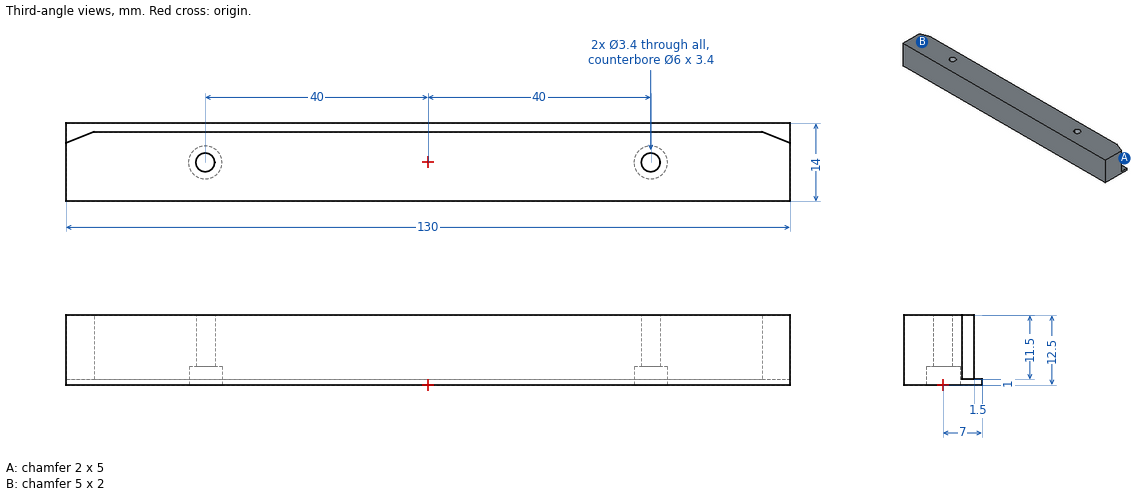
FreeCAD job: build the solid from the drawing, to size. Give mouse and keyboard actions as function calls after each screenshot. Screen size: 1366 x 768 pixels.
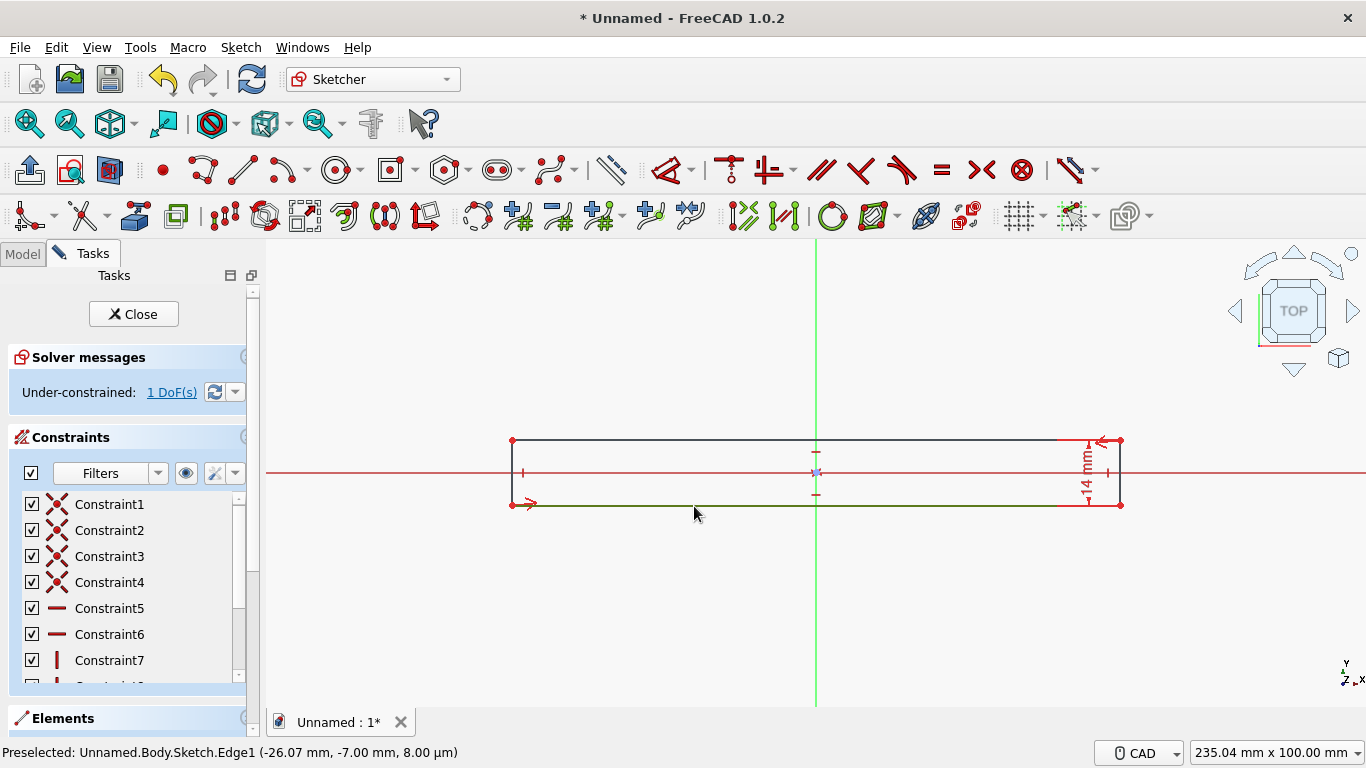
key(l)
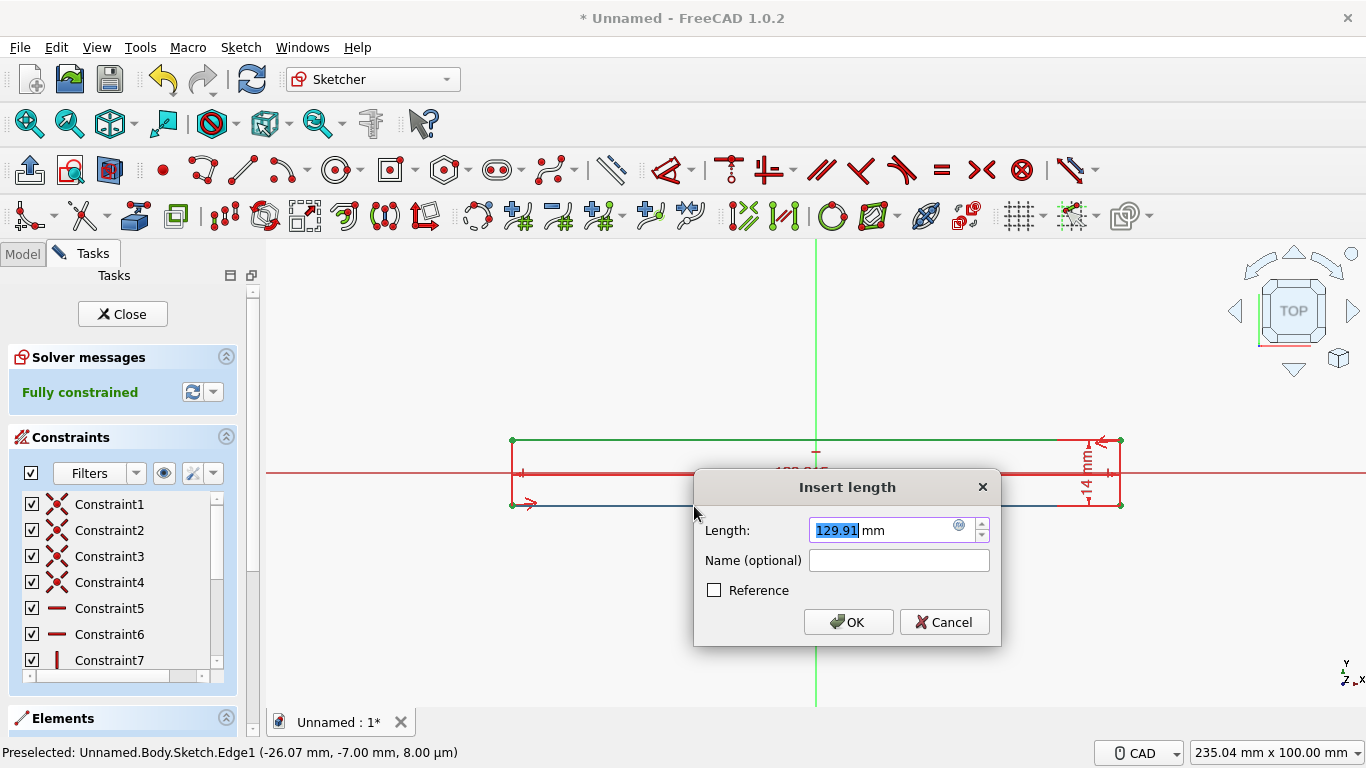
text(130)
key(Return)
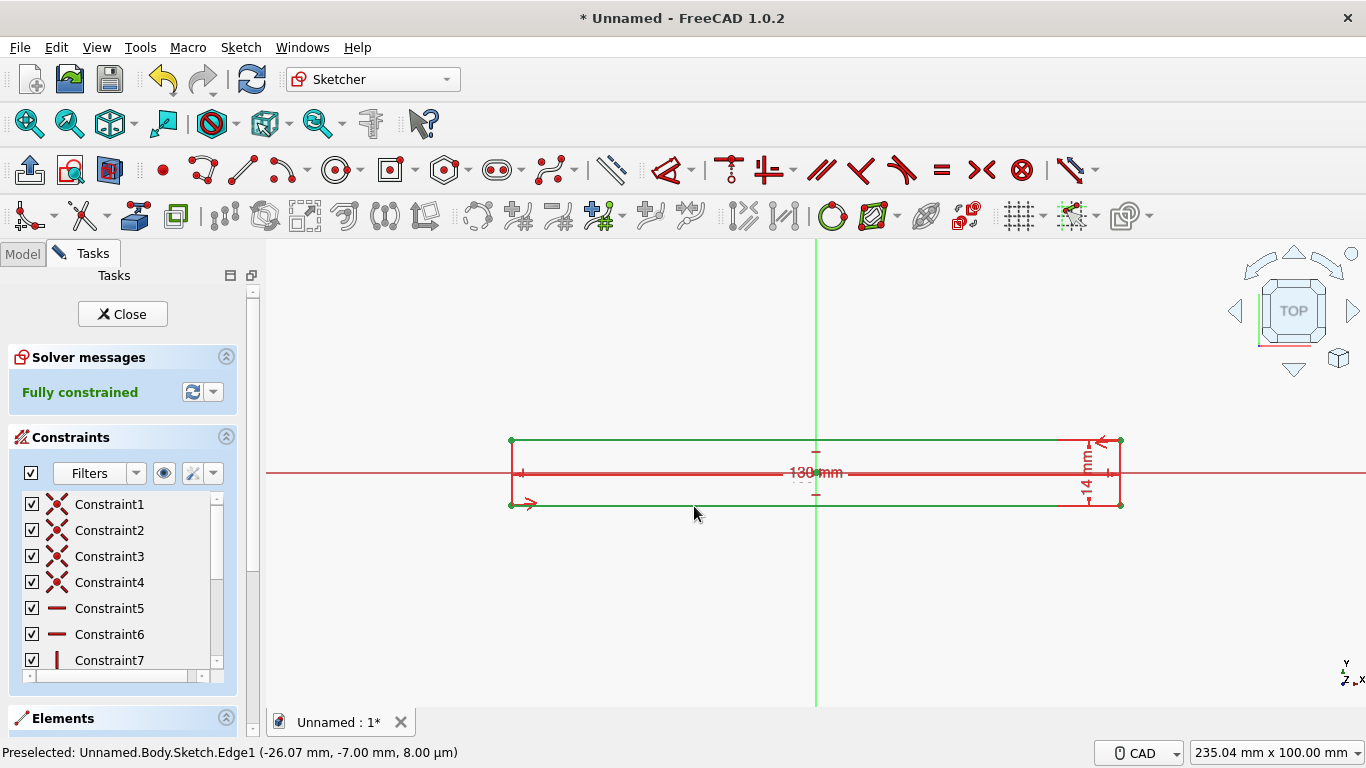
click(123, 314)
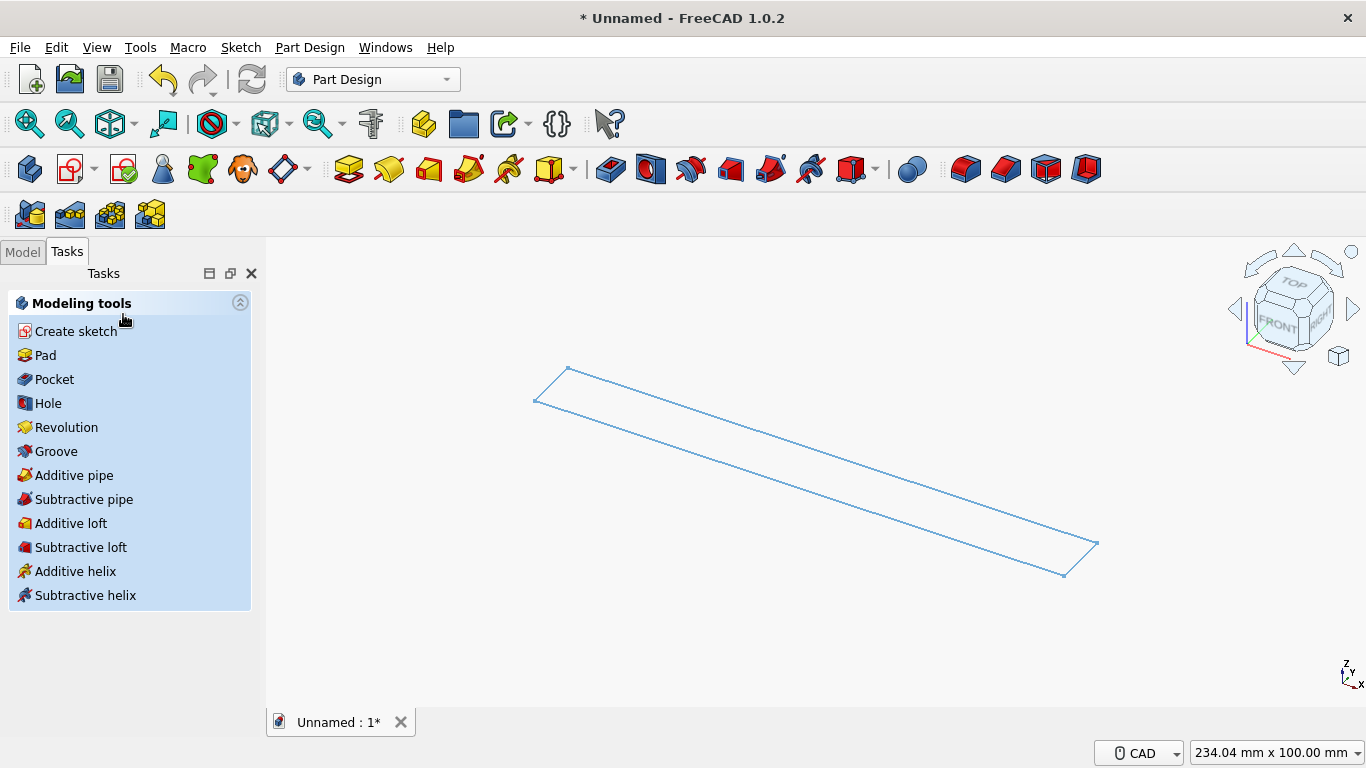
click(350, 170)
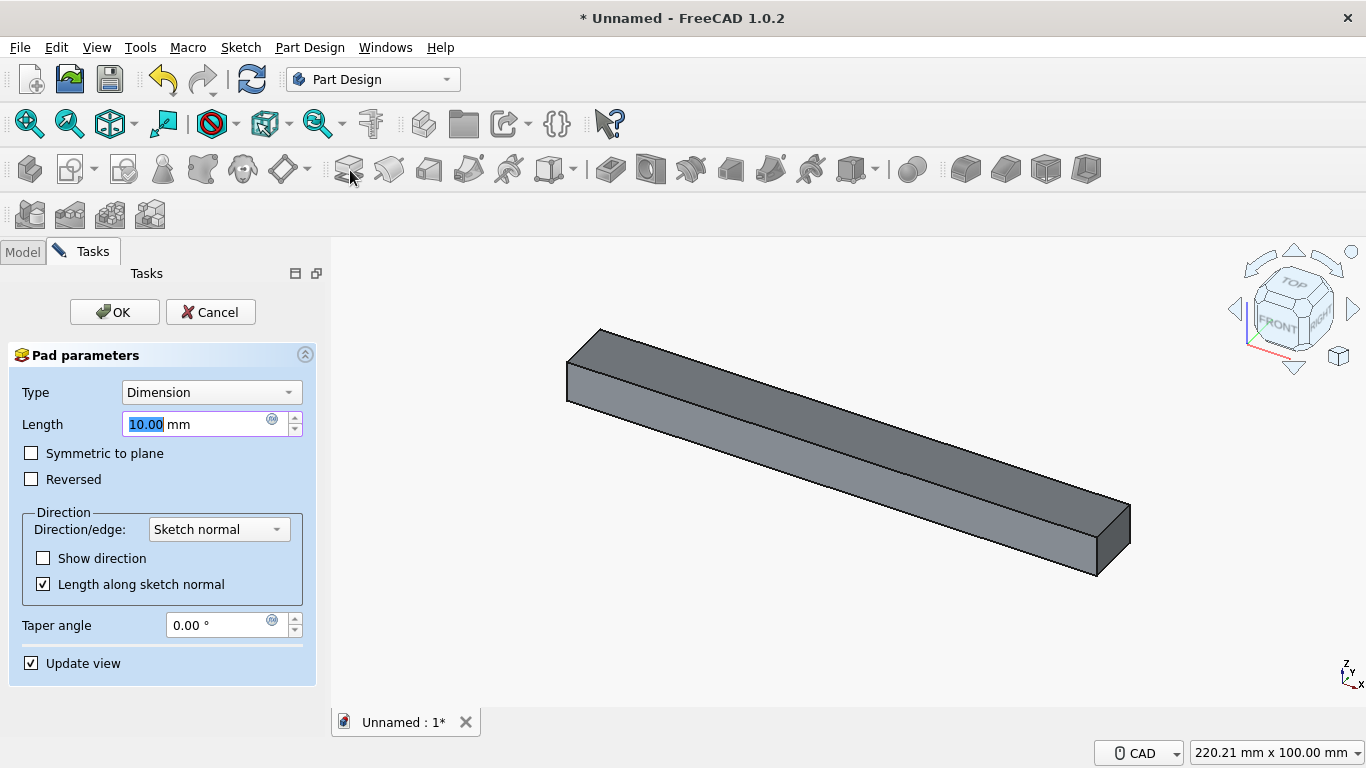
text(12.5)
key(Tab)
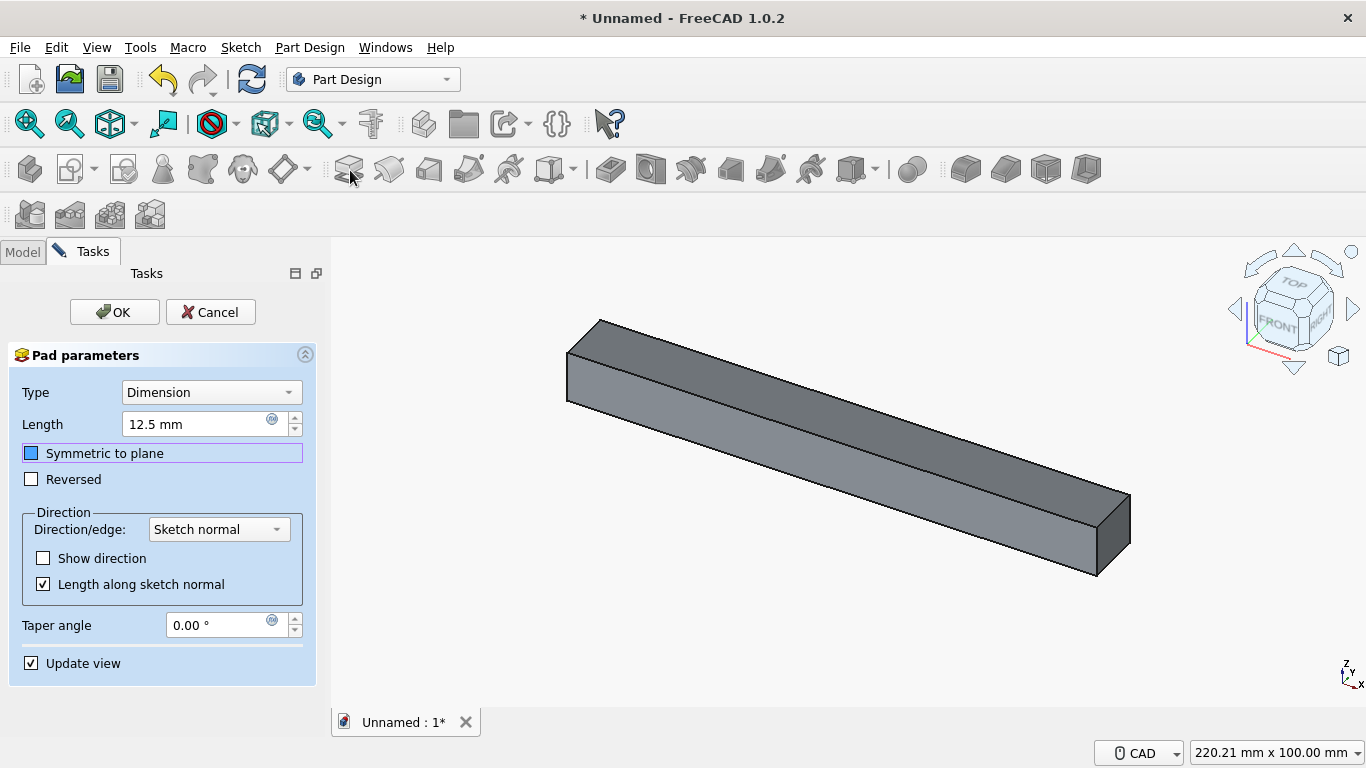
click(115, 312)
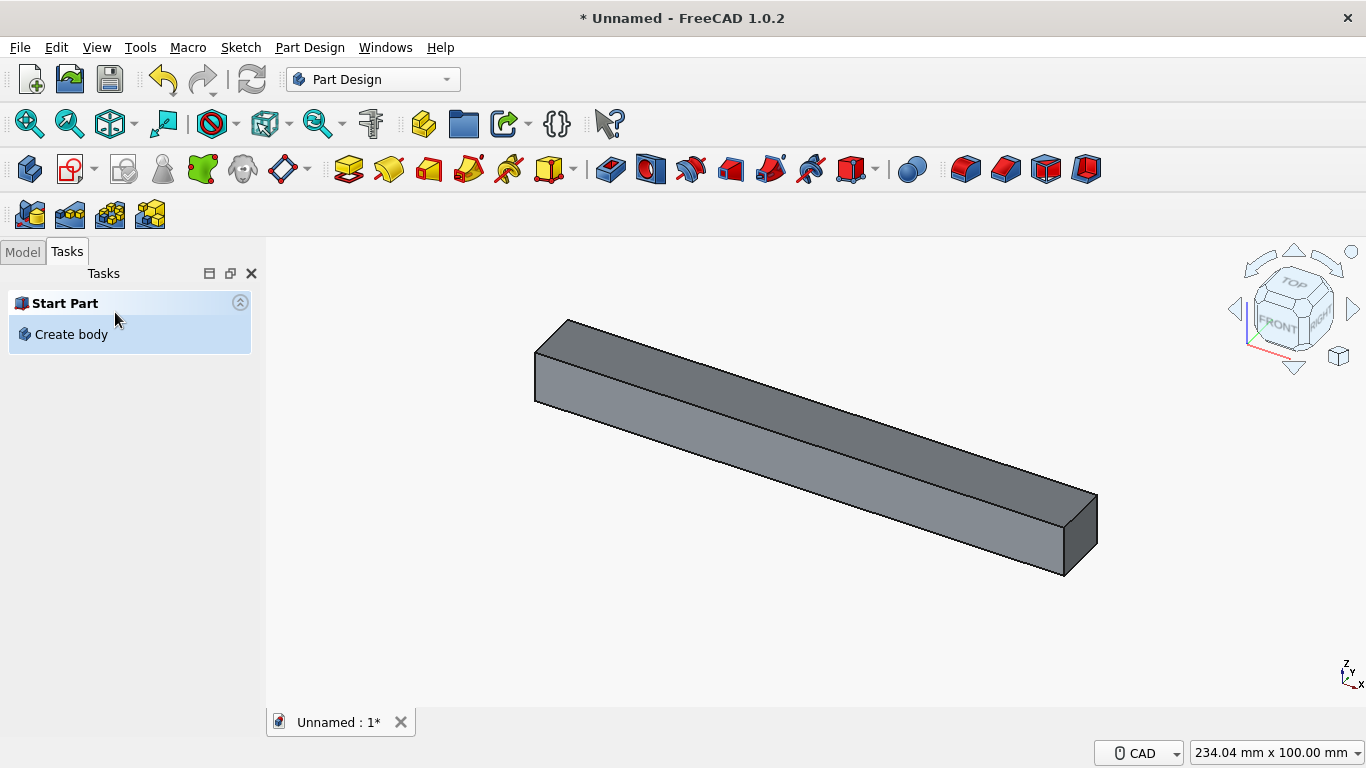
click(1081, 535)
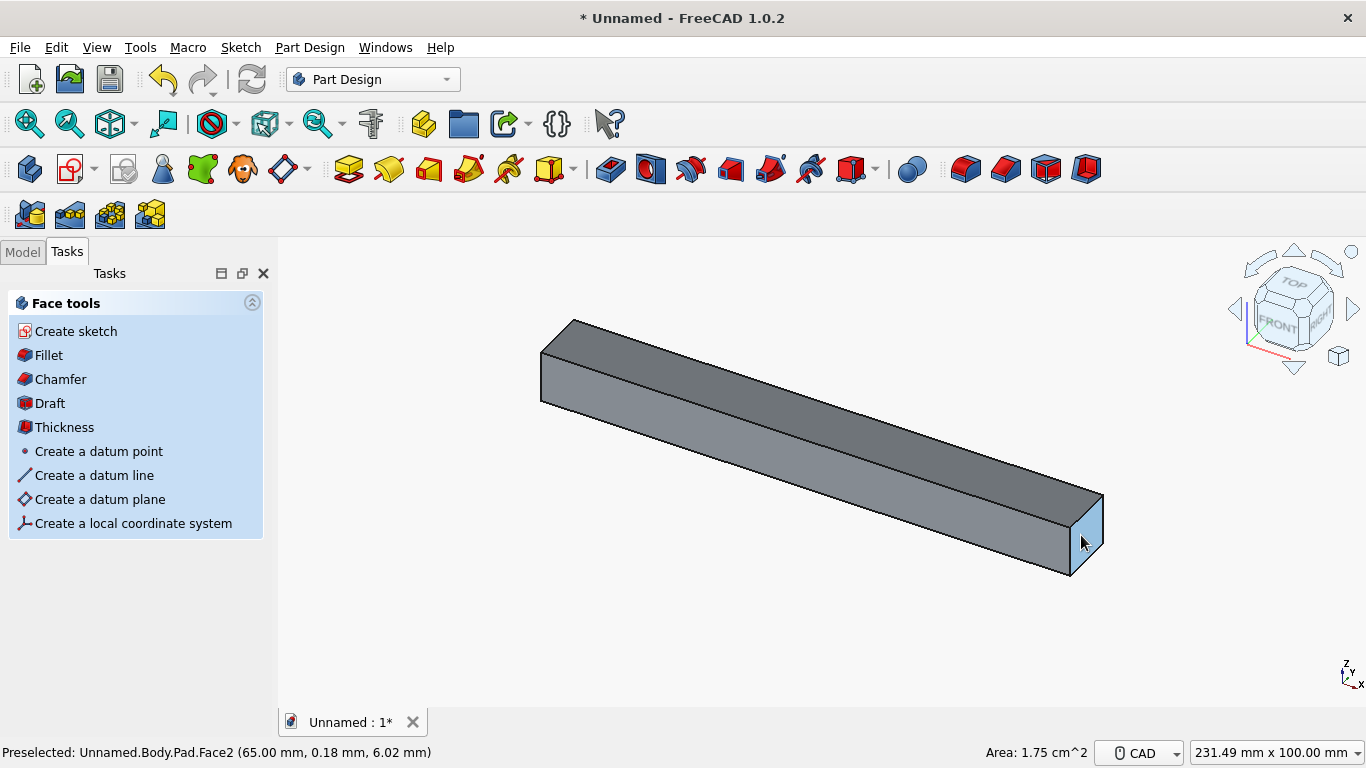
click(70, 170)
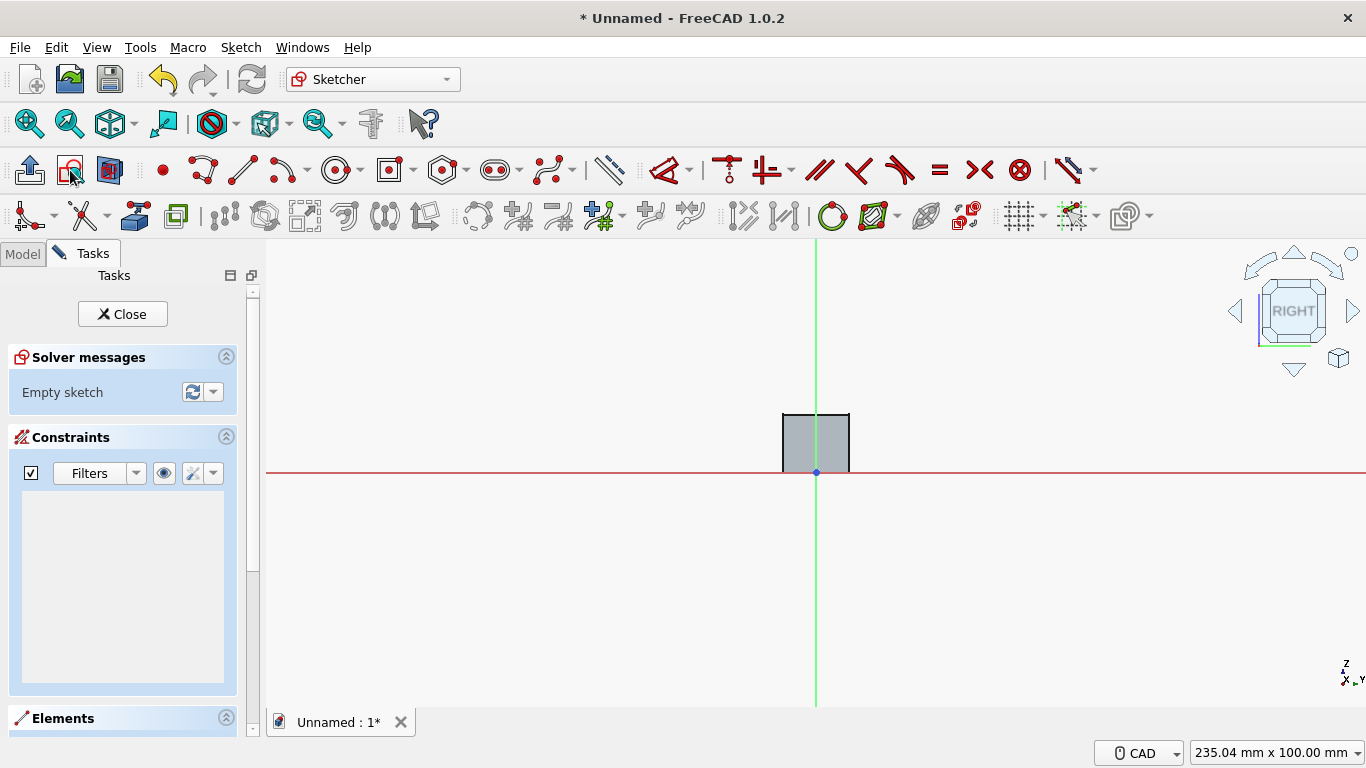
scroll(854, 436, up, 8)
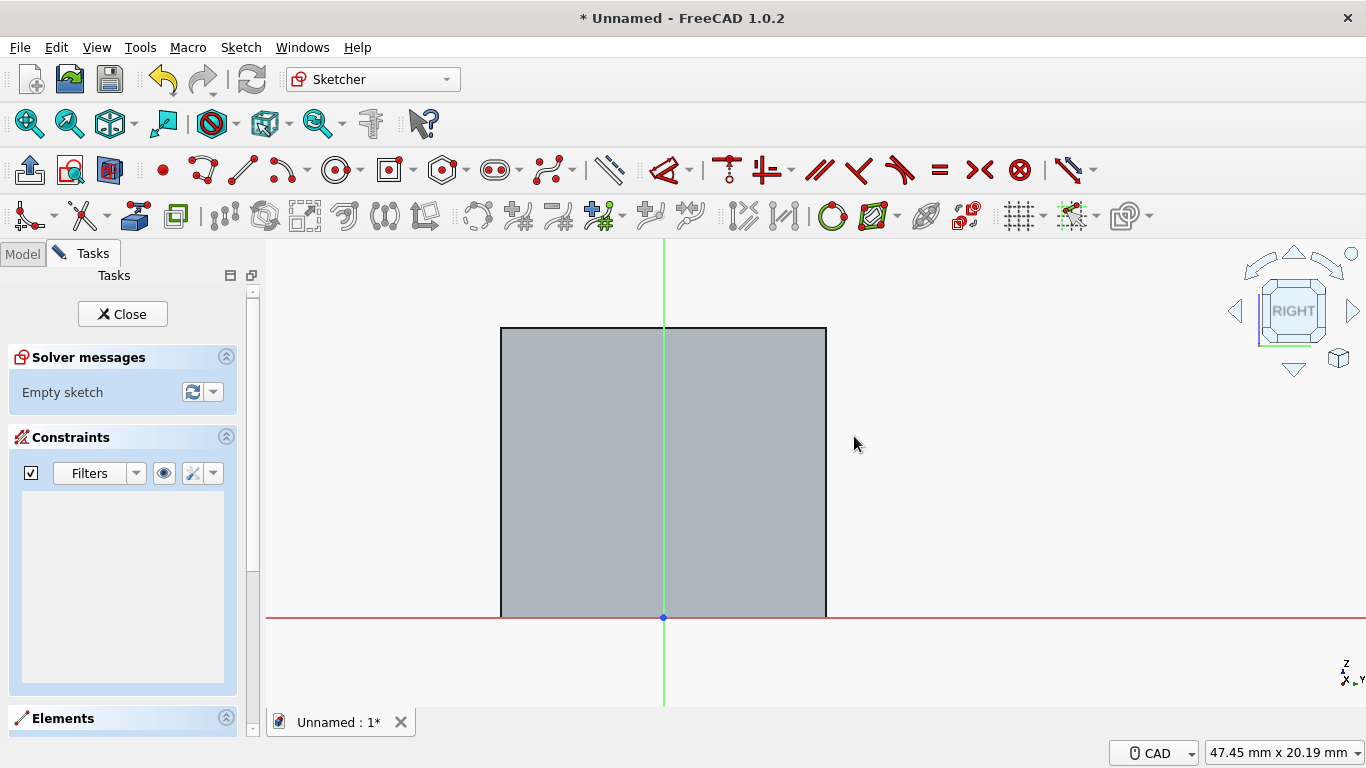
click(416, 170)